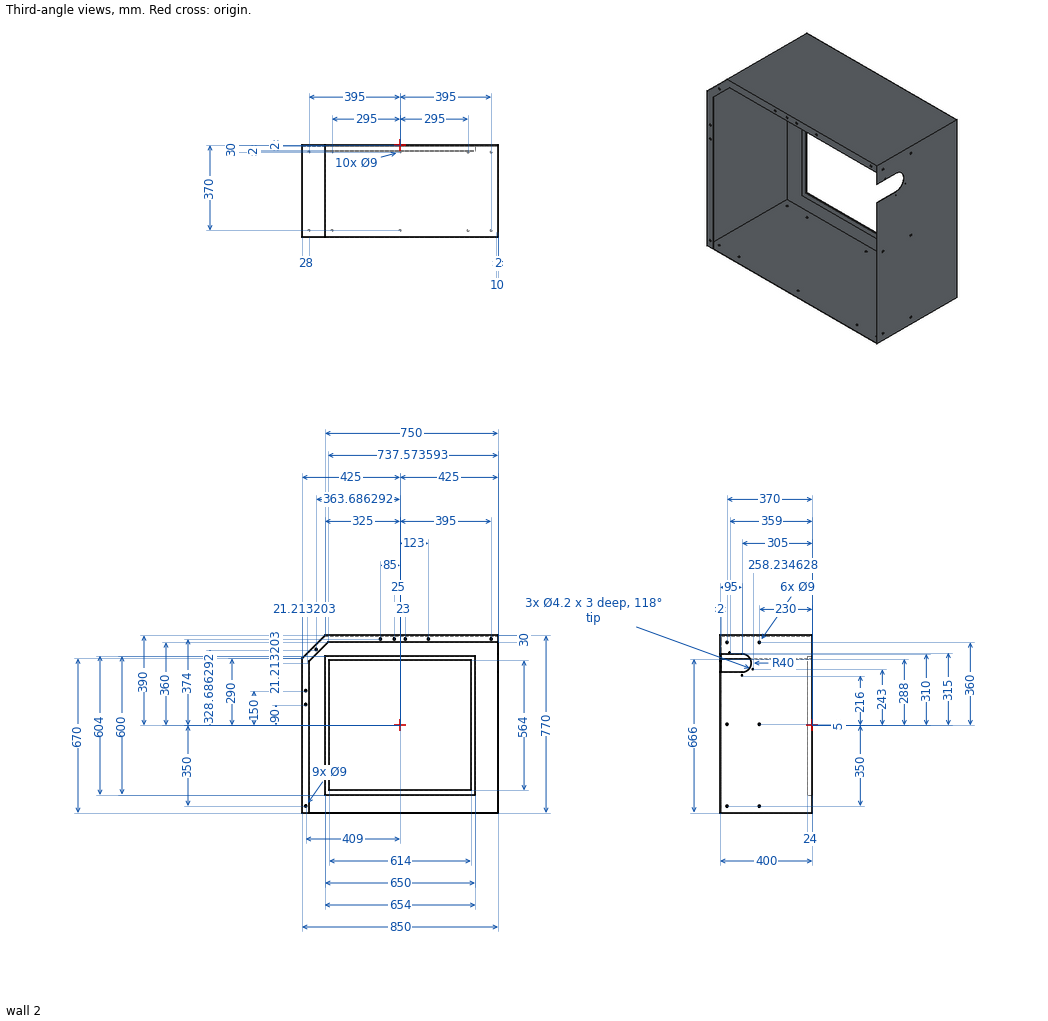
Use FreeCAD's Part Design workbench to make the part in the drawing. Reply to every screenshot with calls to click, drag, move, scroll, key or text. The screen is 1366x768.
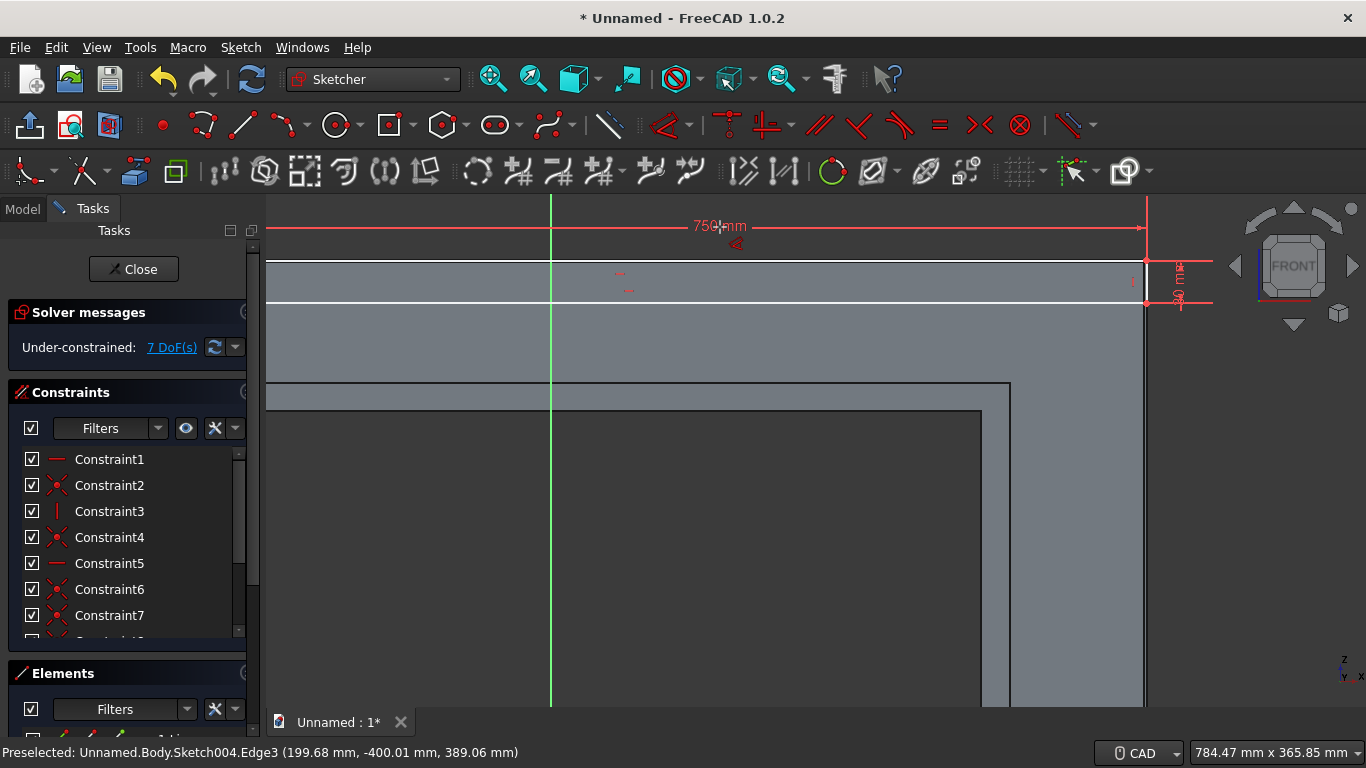
scroll(987, 350, down, 3)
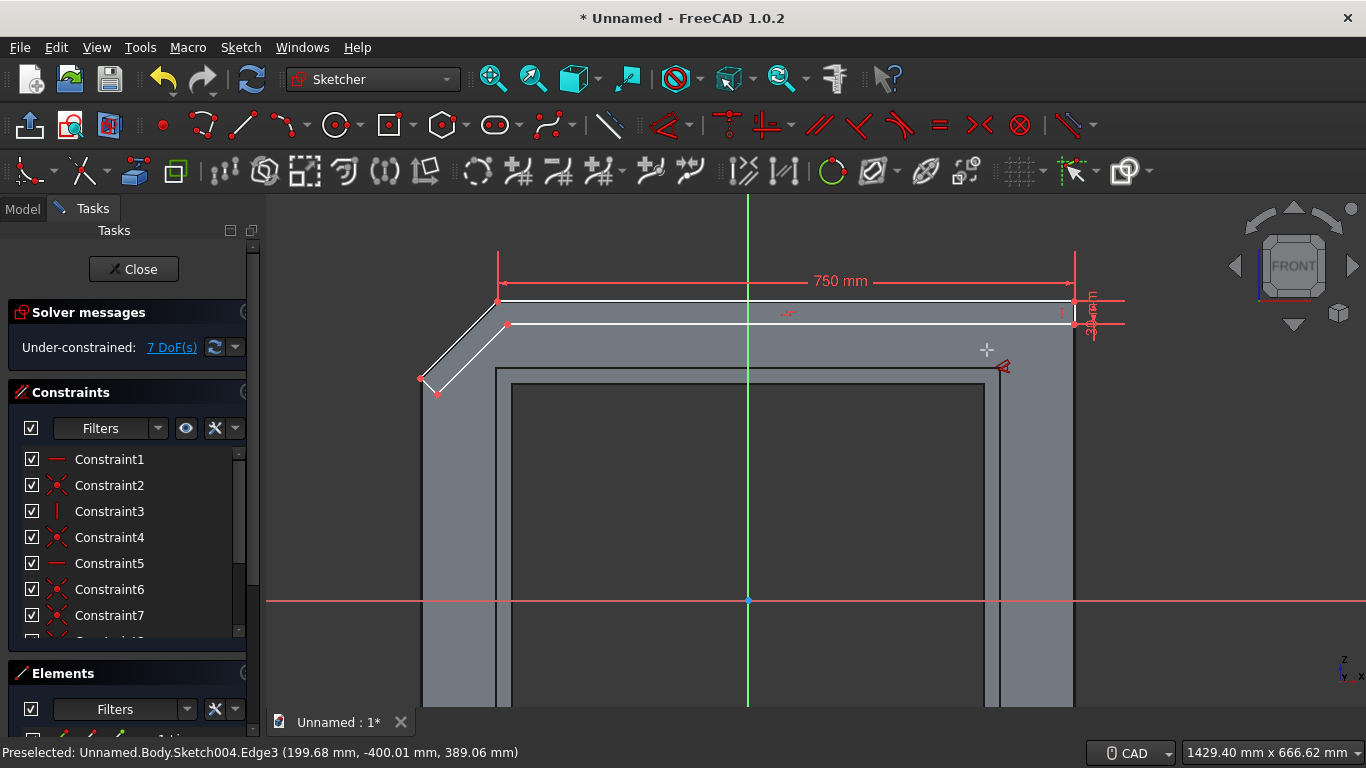
click(508, 324)
click(474, 463)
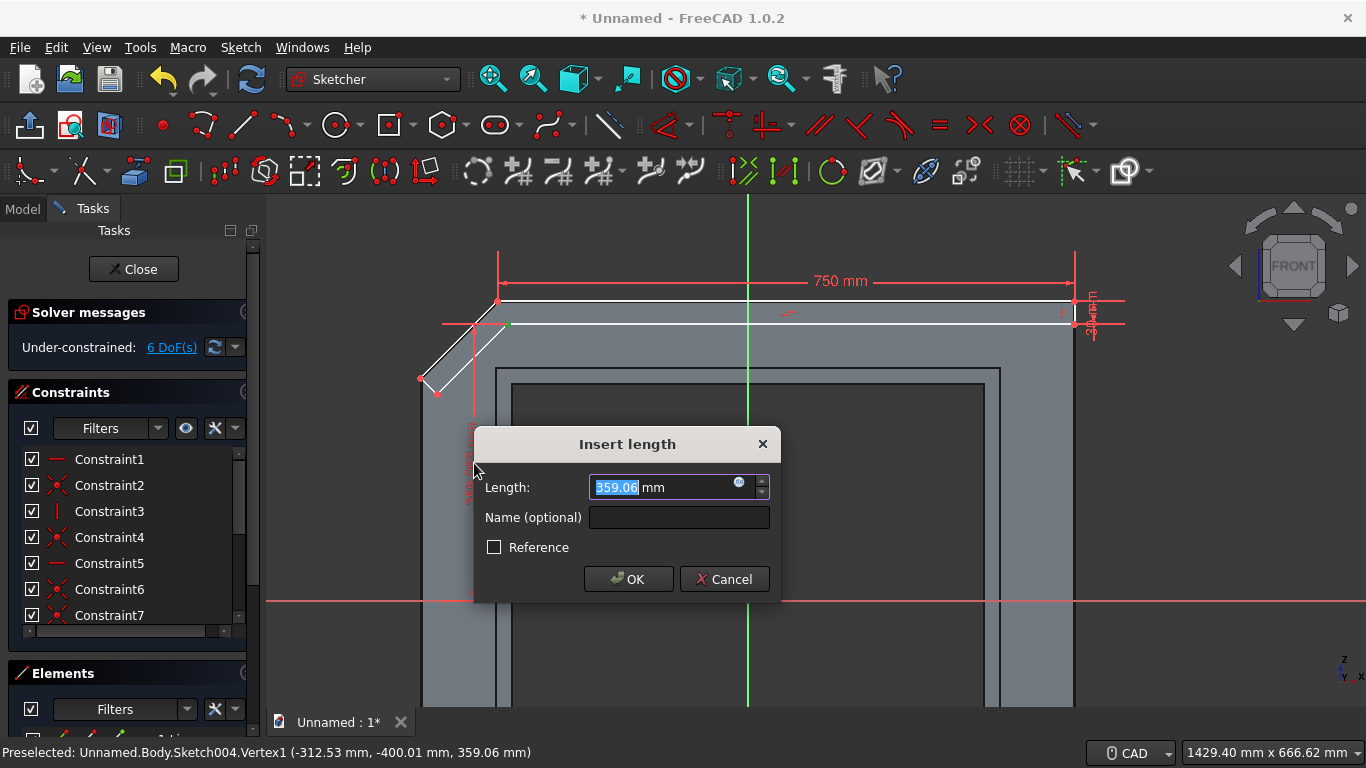
text(360)
key(Return)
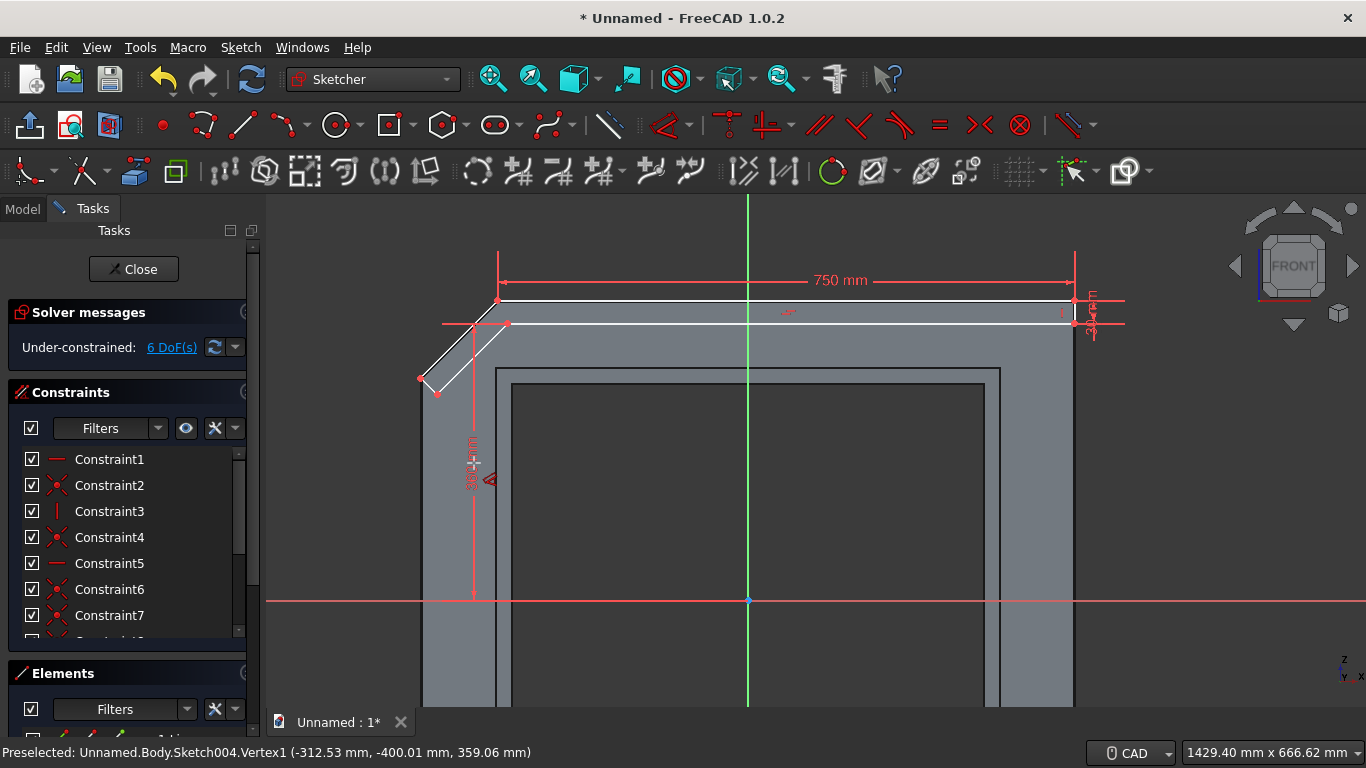
click(1075, 324)
click(911, 635)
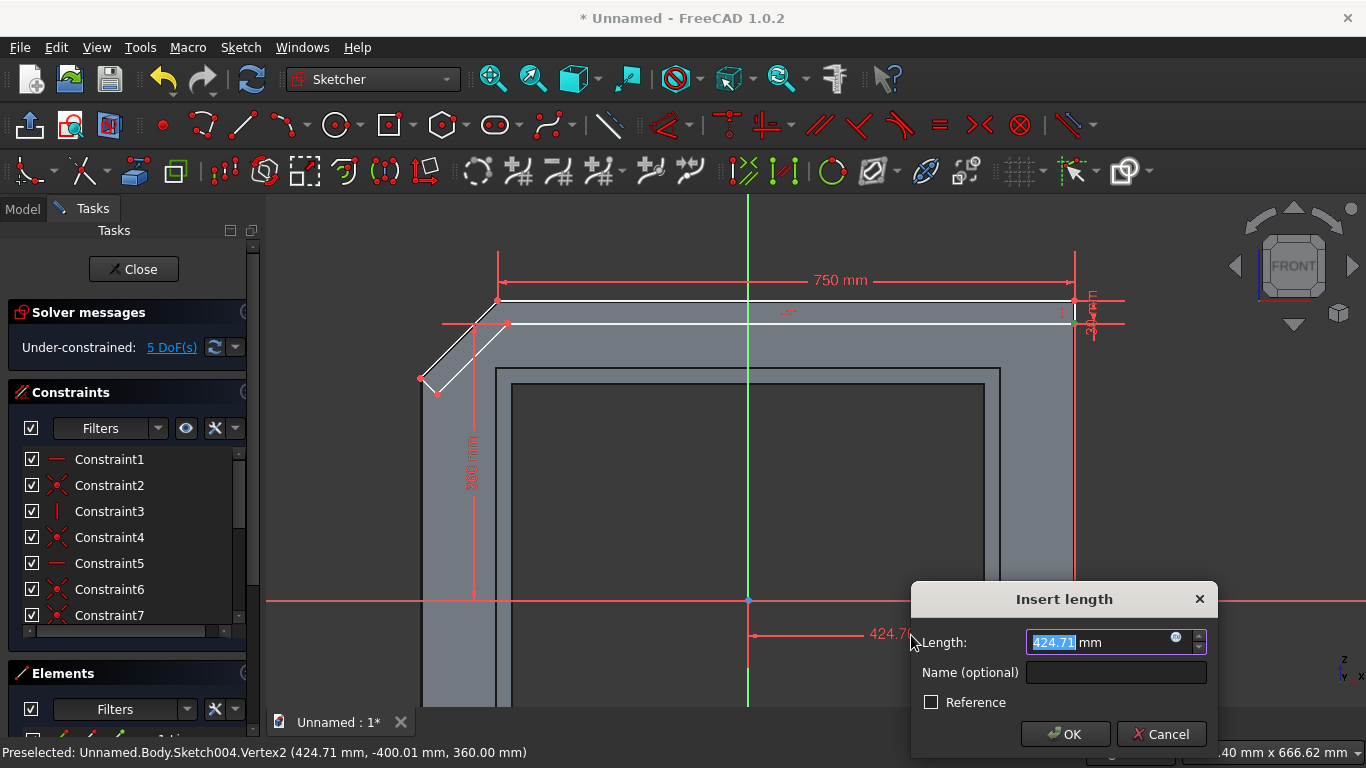
text(425)
key(Return)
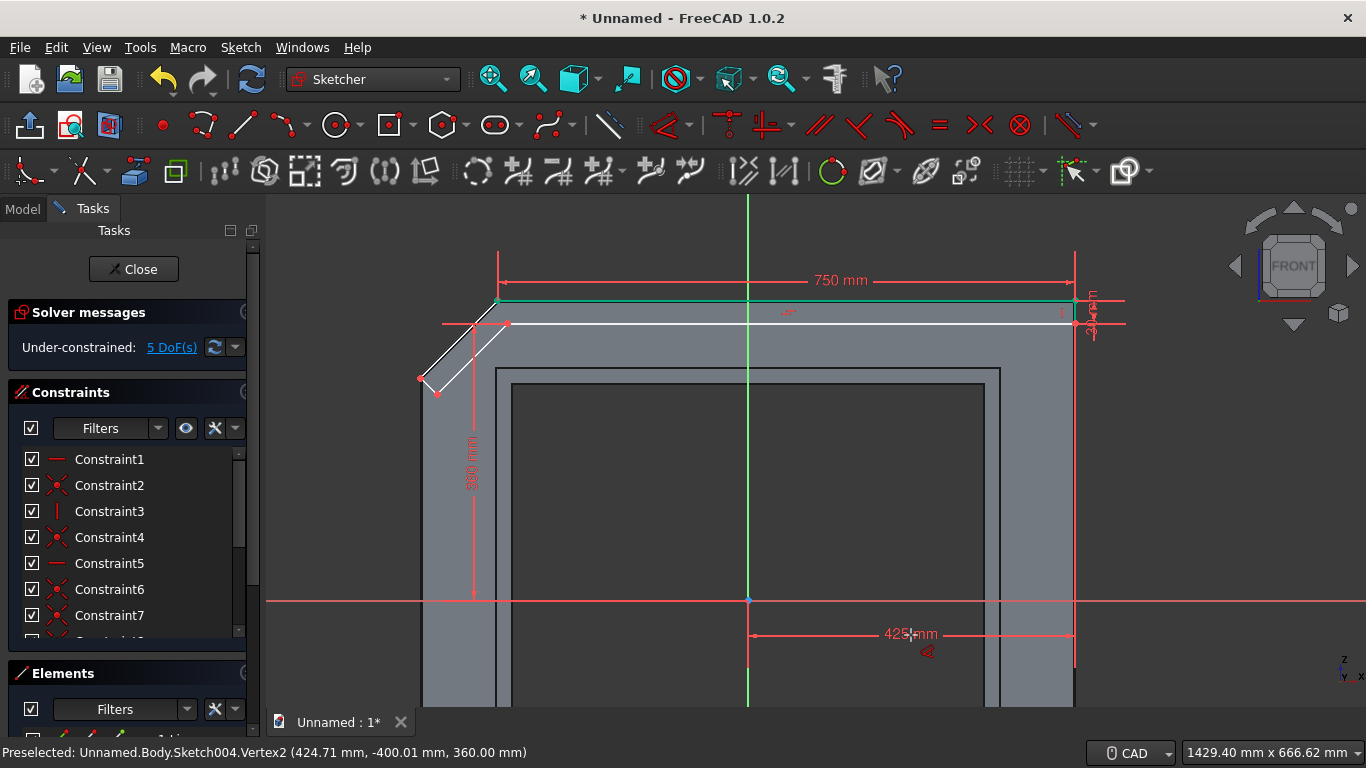
click(421, 378)
click(584, 635)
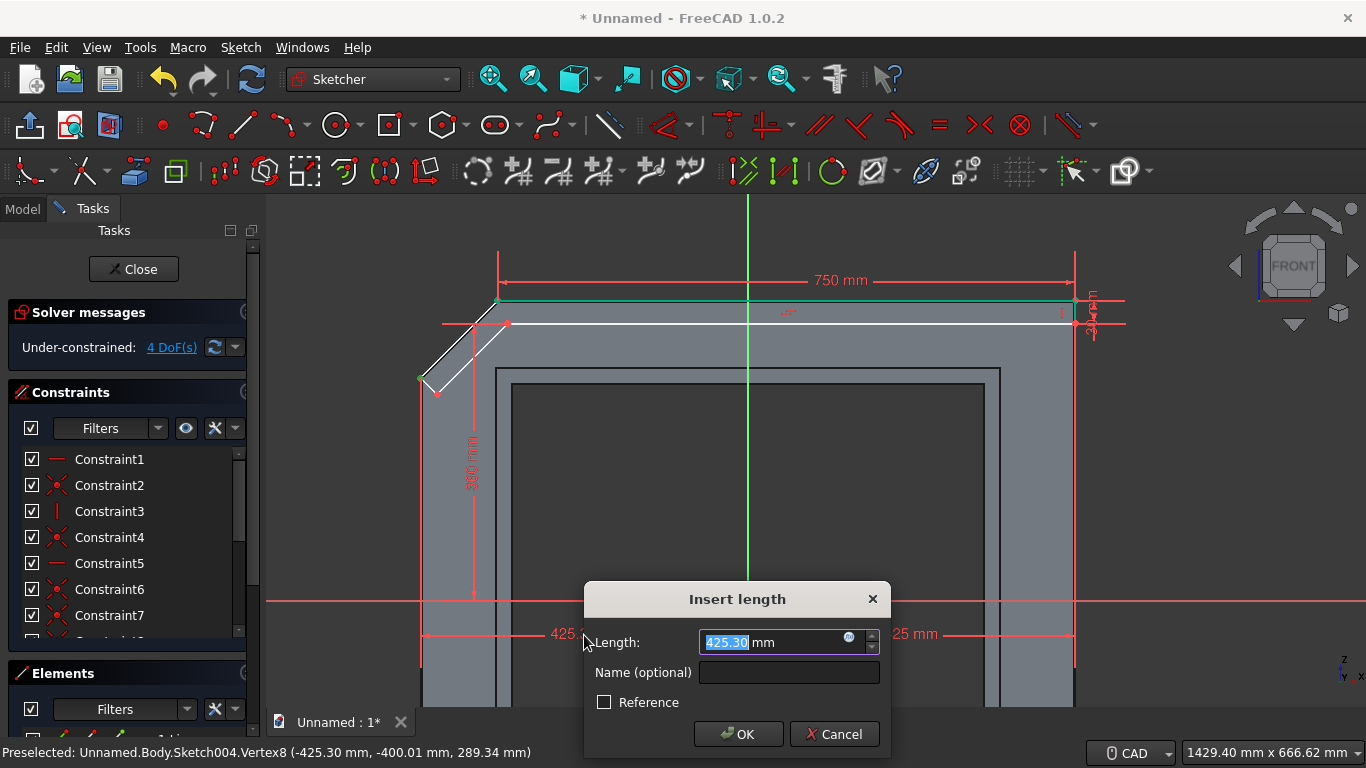
text(425)
key(Return)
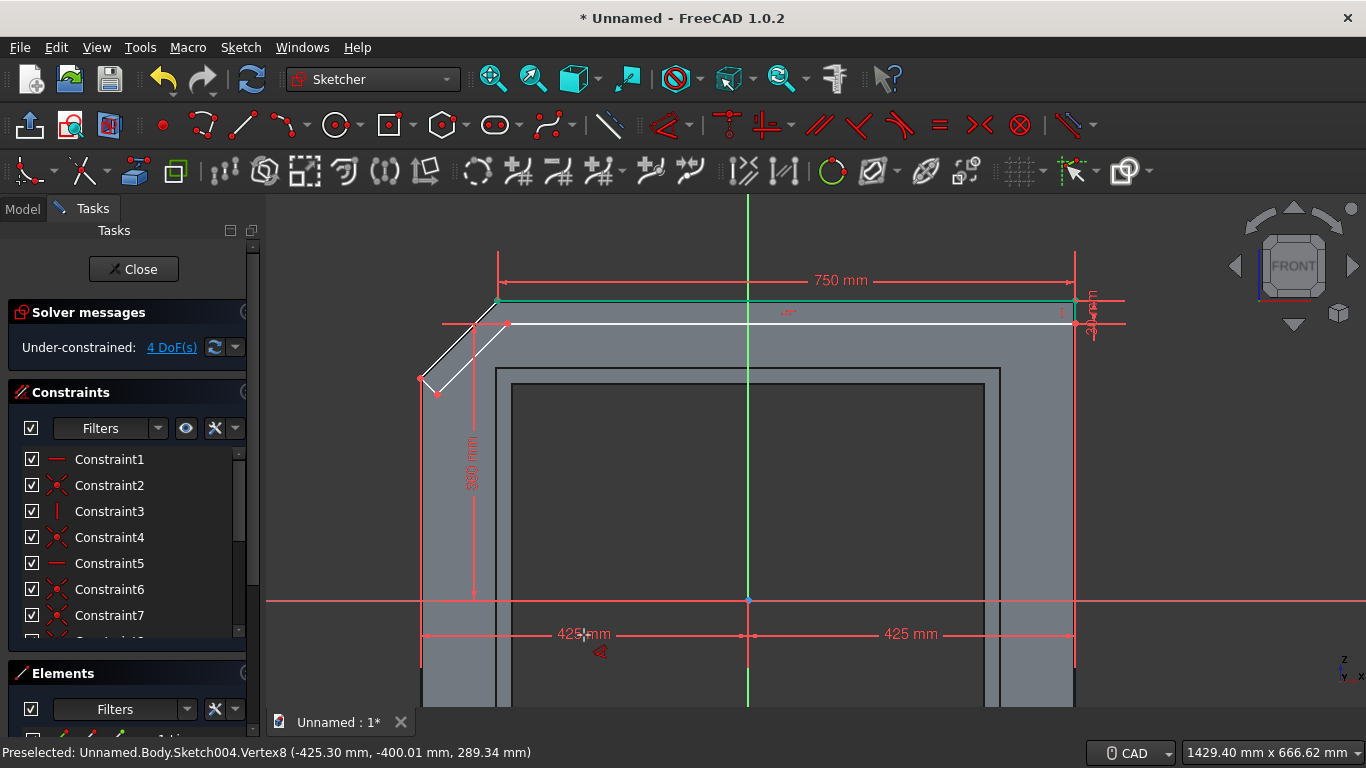
click(421, 378)
click(387, 489)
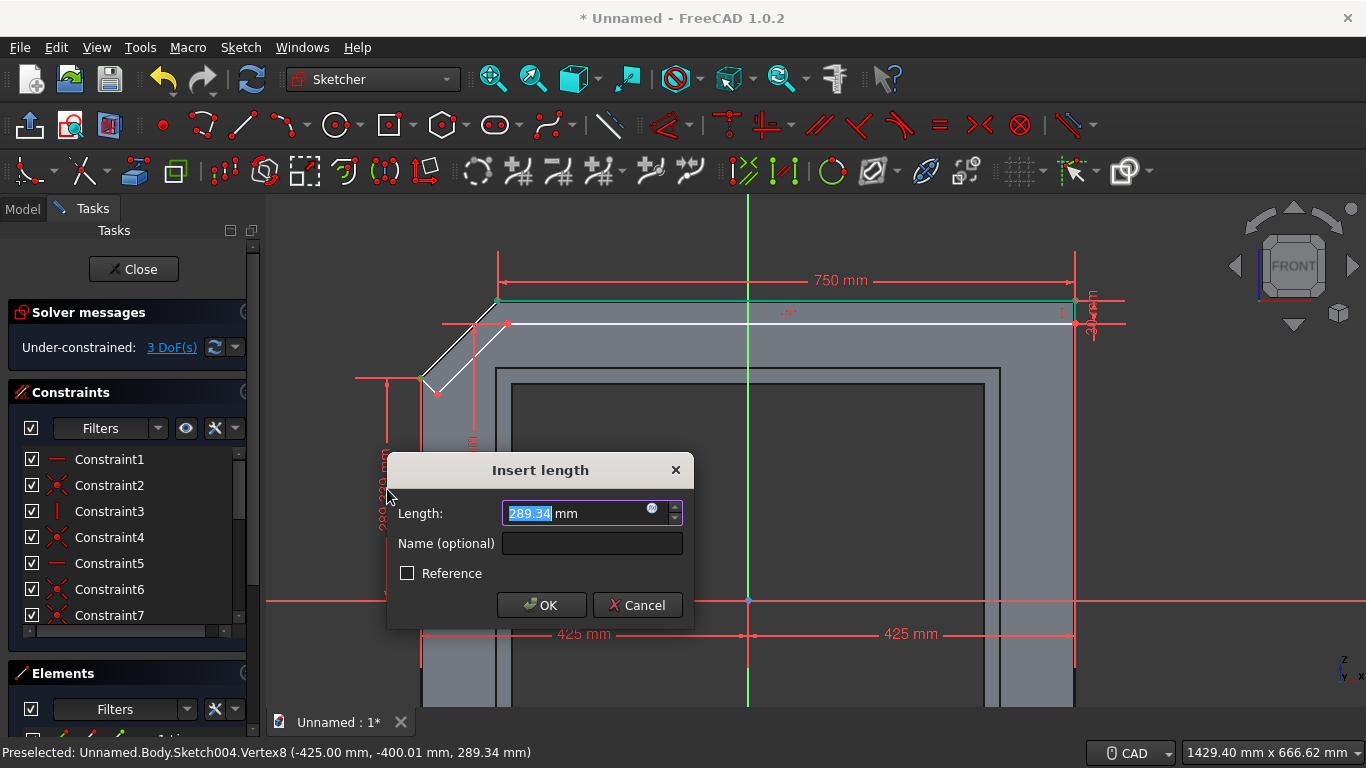
text(290)
key(Return)